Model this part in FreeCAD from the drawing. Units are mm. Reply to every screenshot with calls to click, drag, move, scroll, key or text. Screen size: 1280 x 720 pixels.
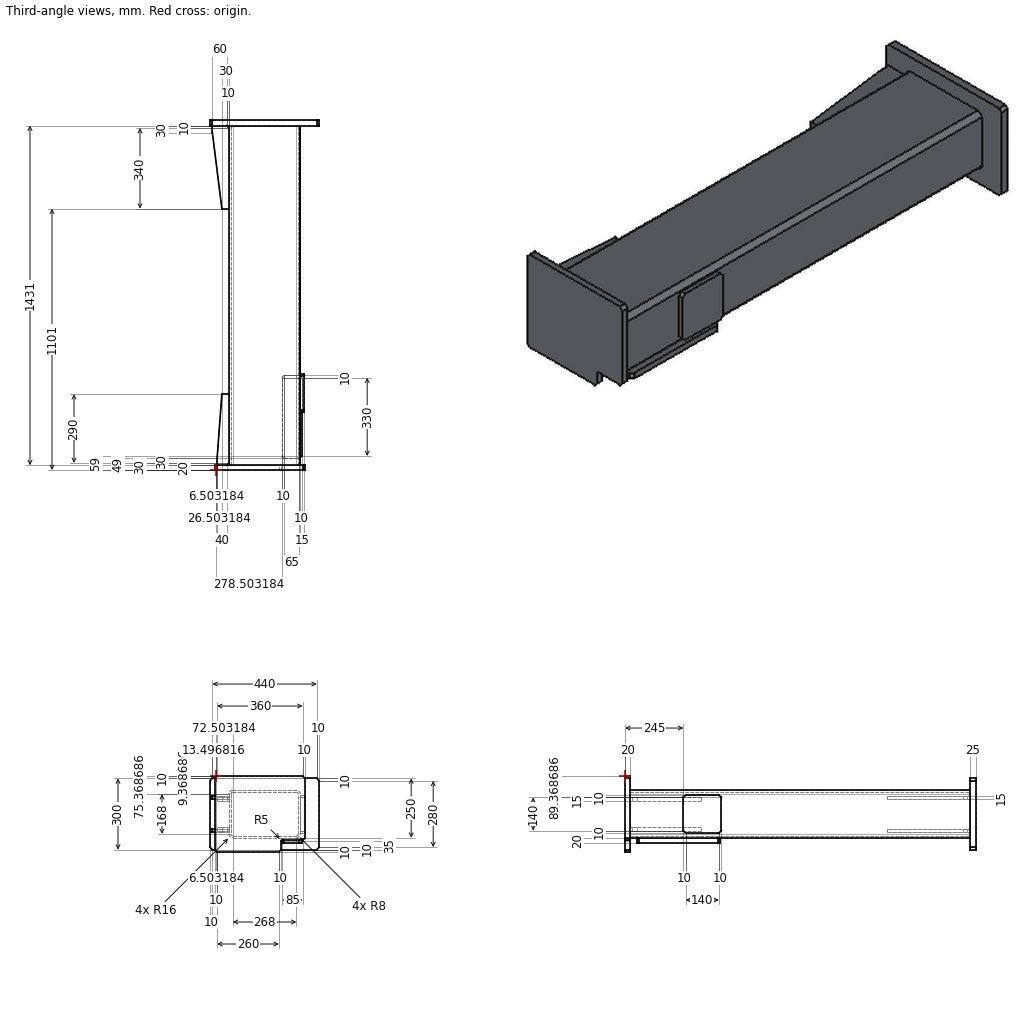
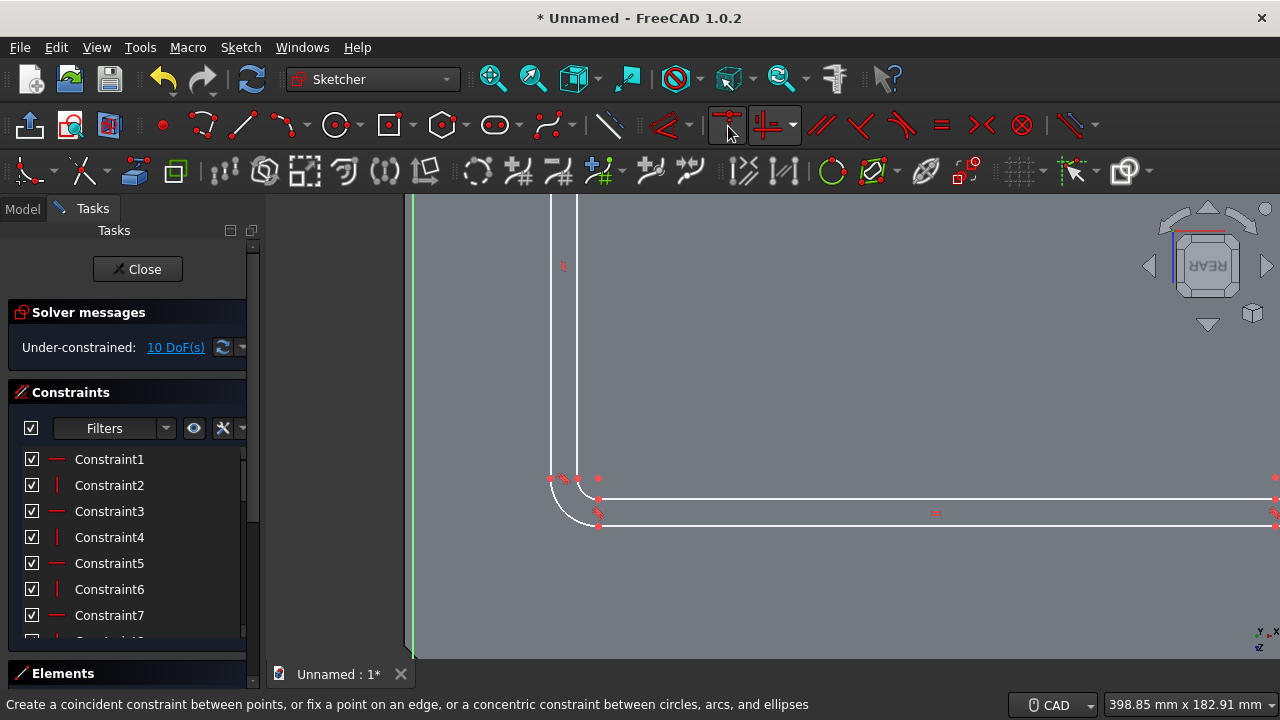
scroll(572, 497, down, 4)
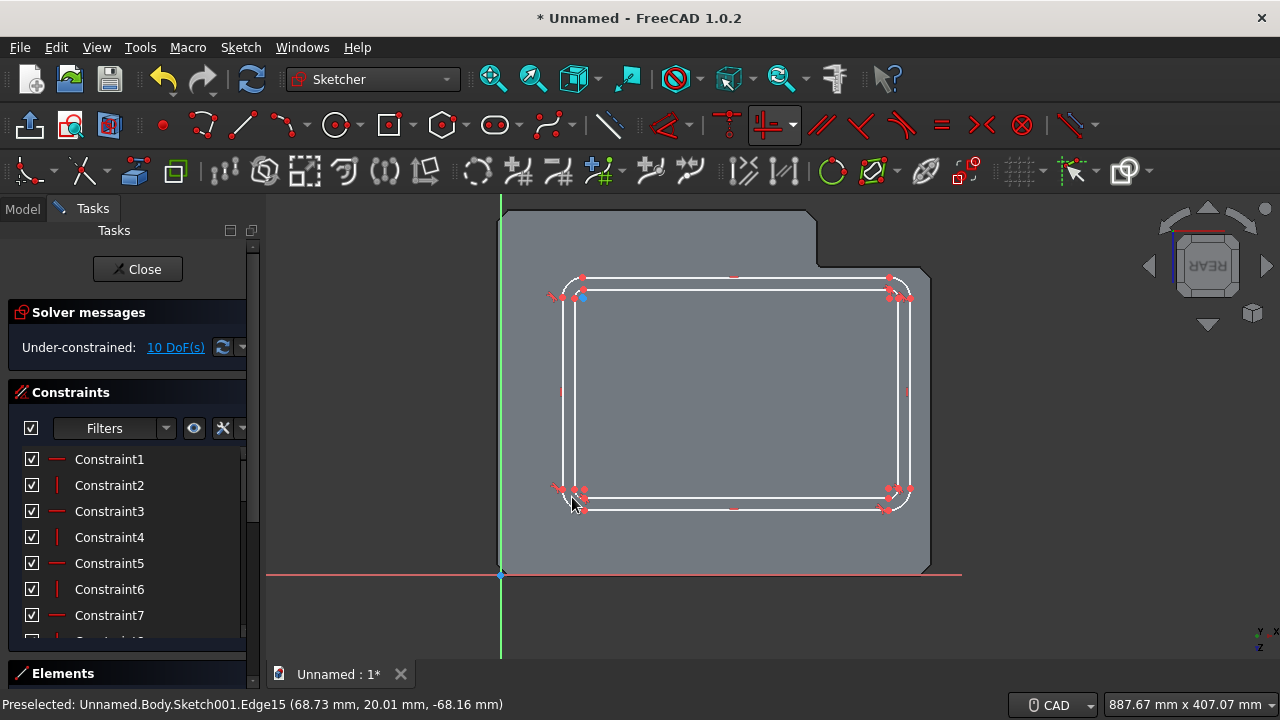
scroll(574, 280, up, 2)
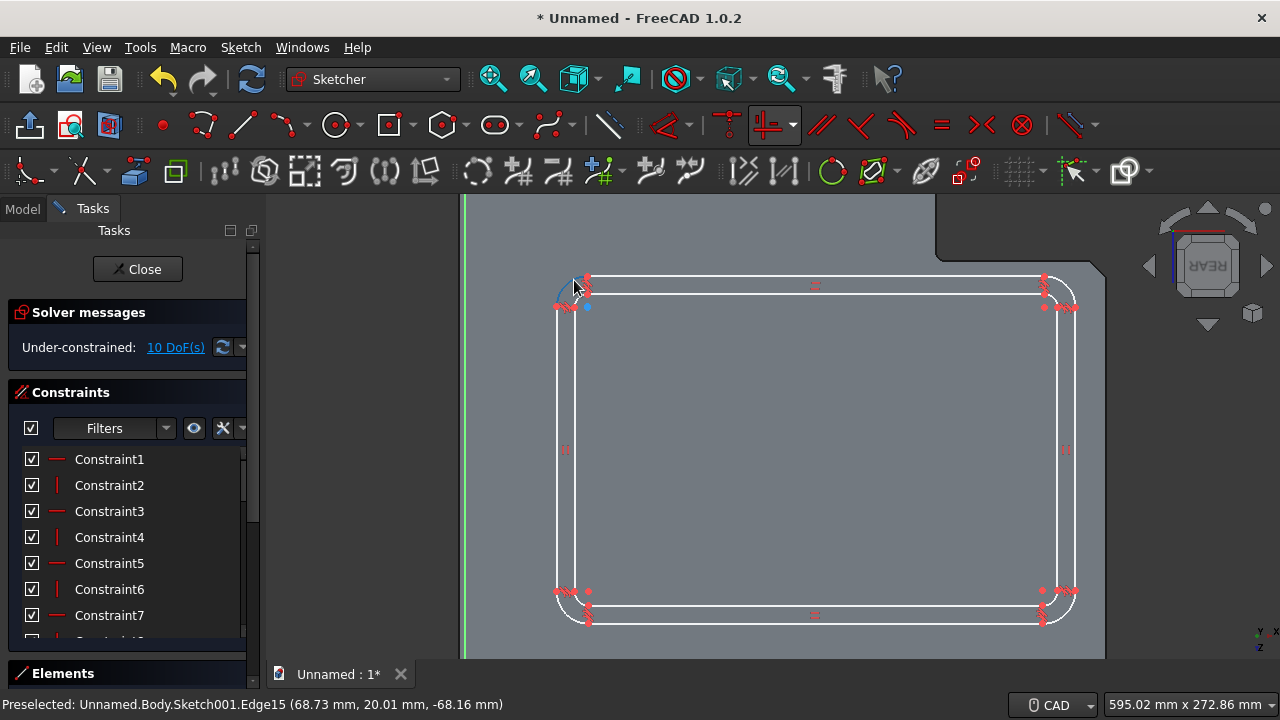
click(573, 280)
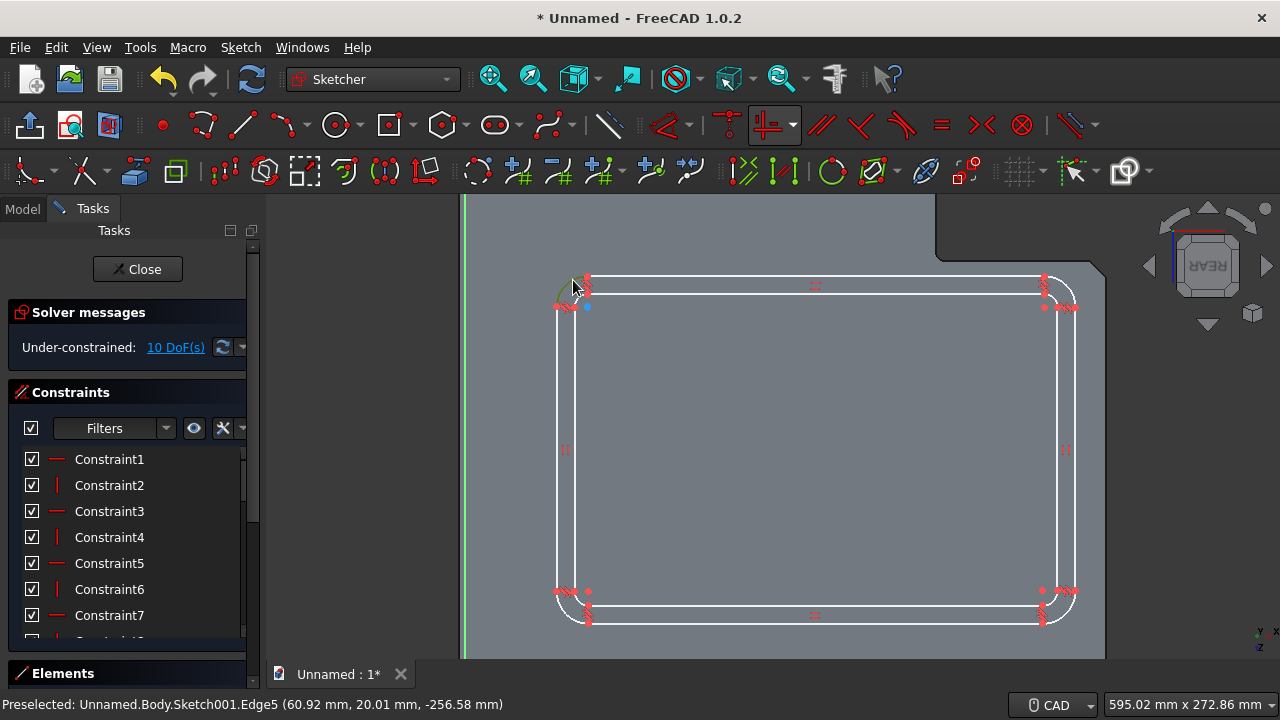
click(560, 606)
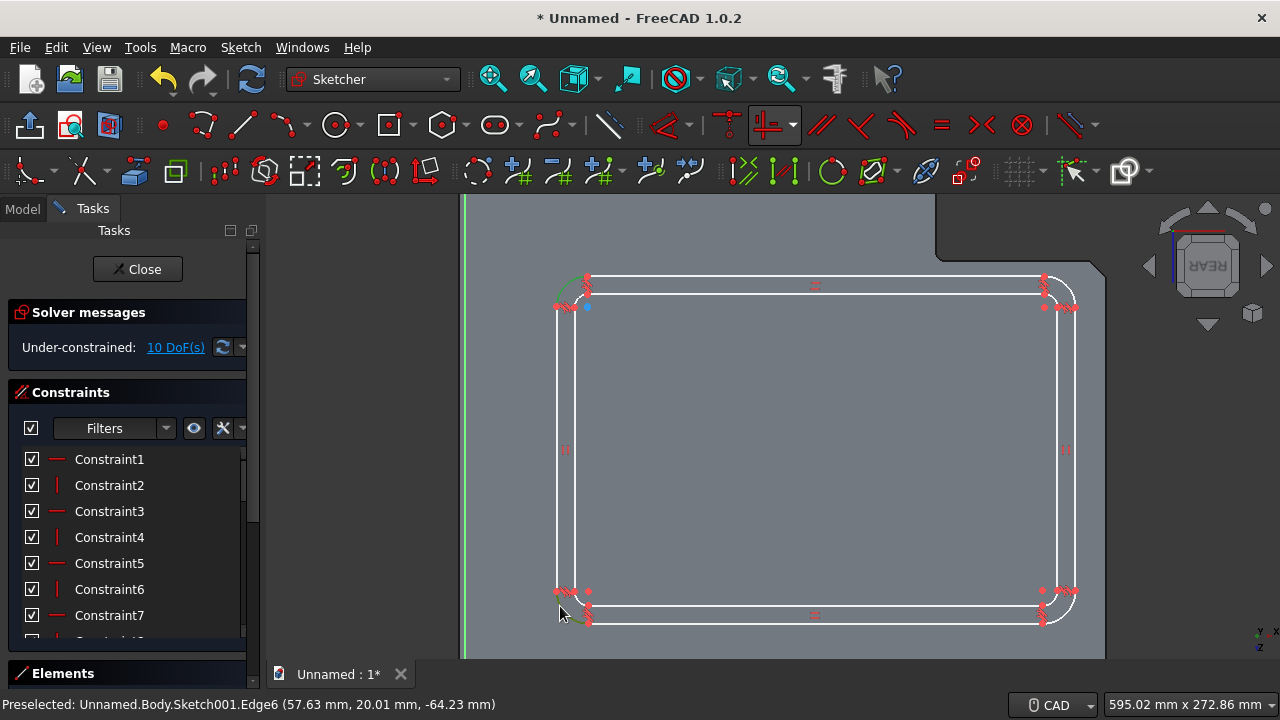
click(1058, 620)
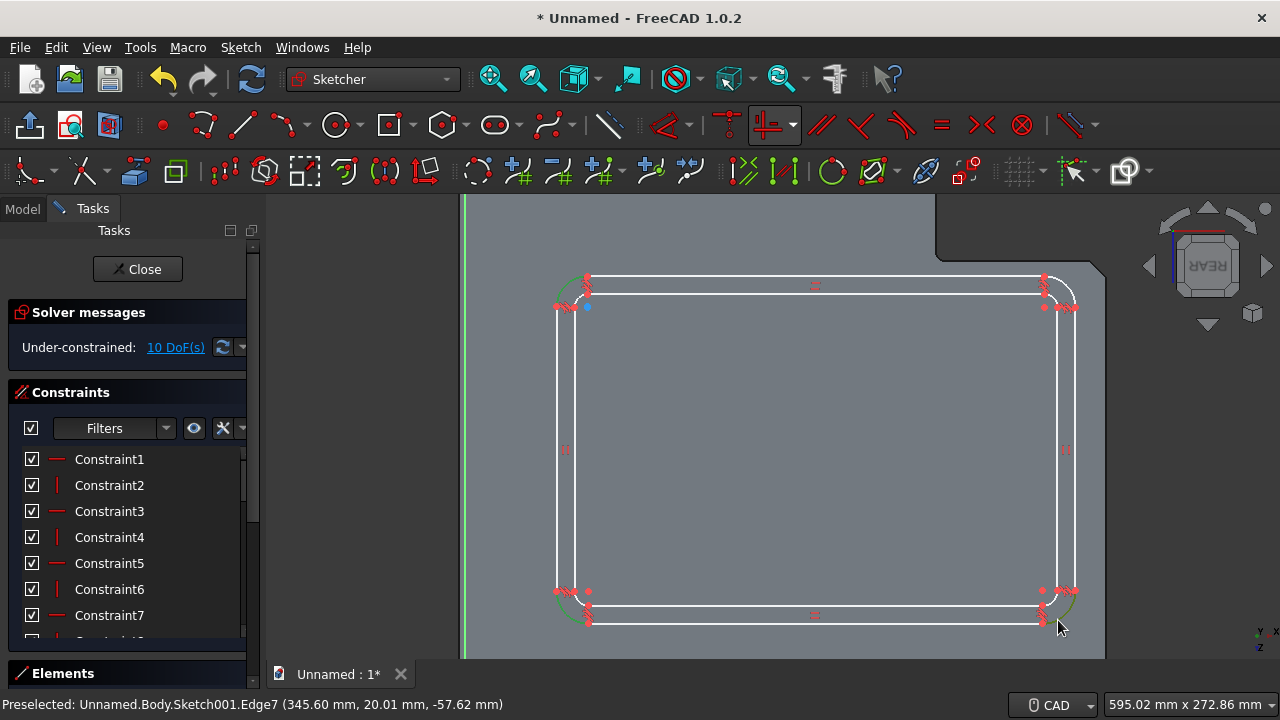
click(1072, 293)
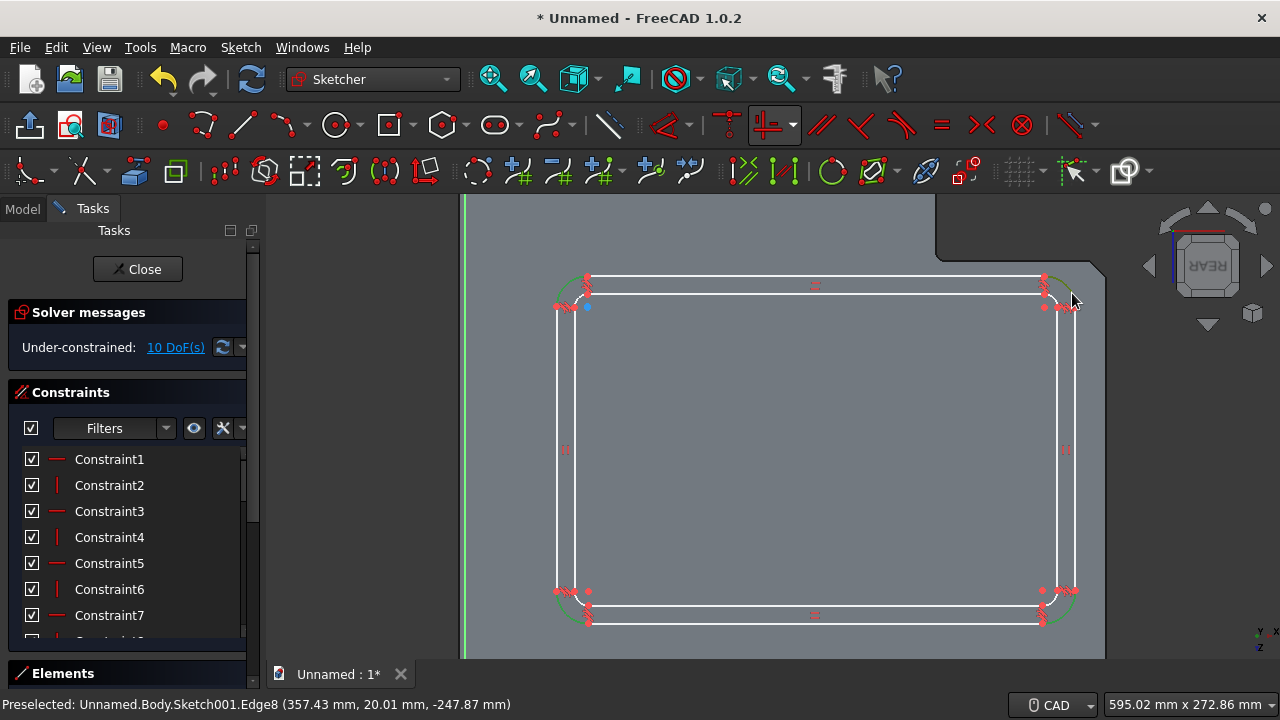
key(e)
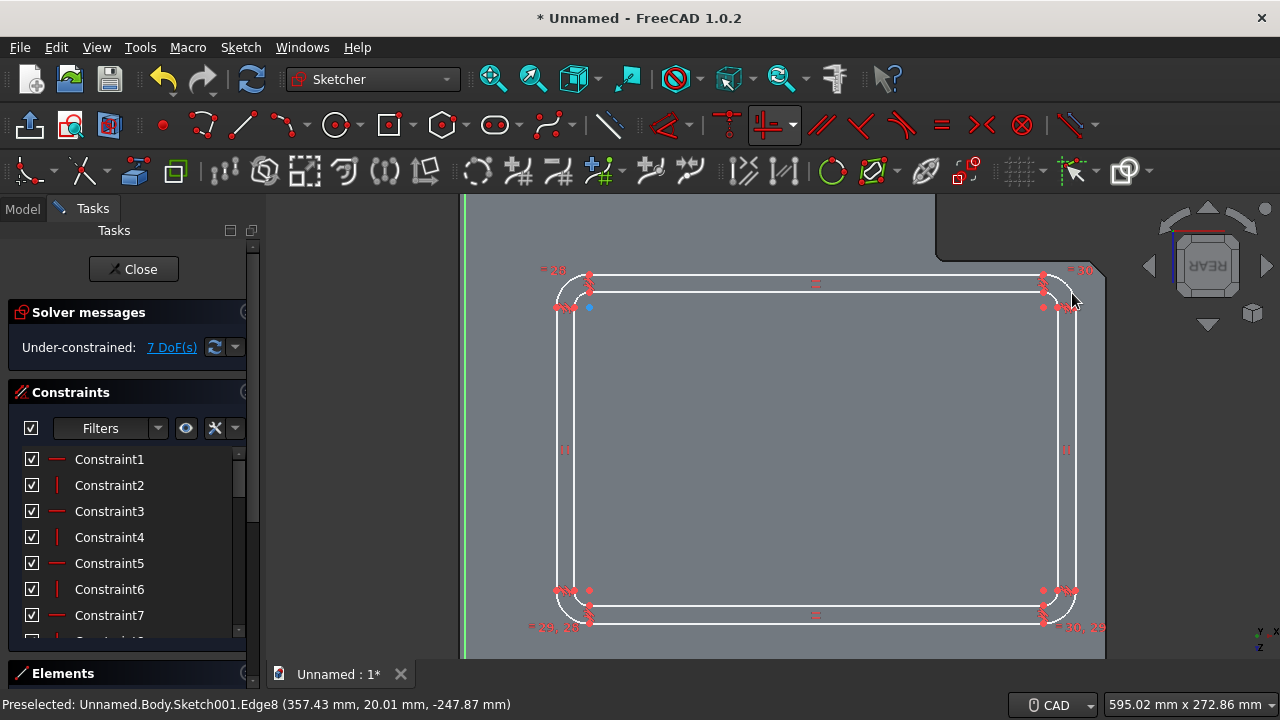
click(1054, 297)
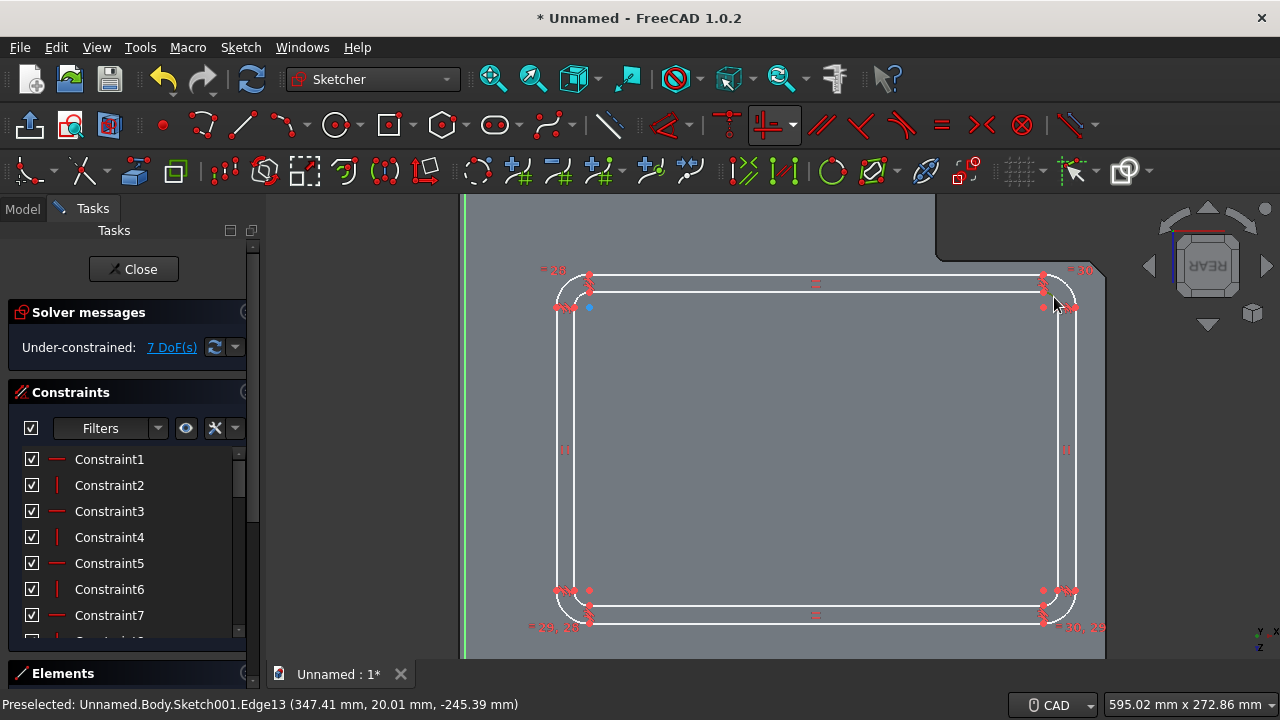
click(579, 297)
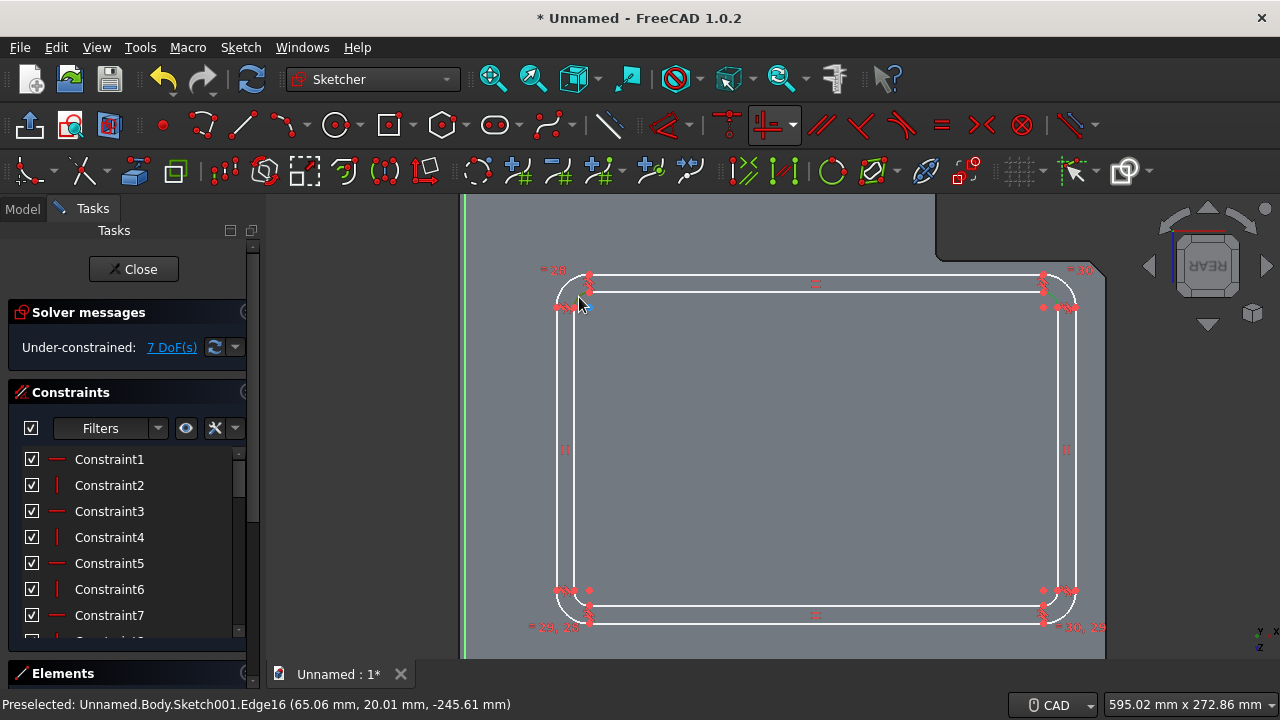
click(942, 126)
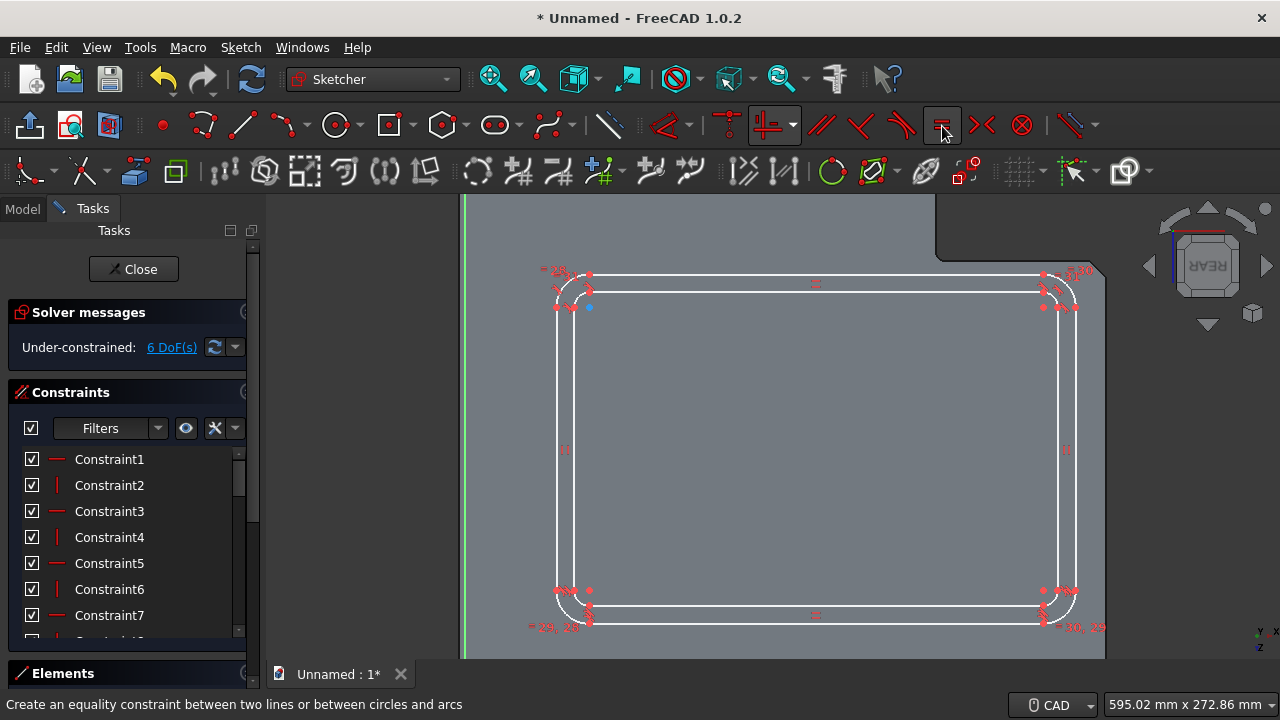
click(664, 126)